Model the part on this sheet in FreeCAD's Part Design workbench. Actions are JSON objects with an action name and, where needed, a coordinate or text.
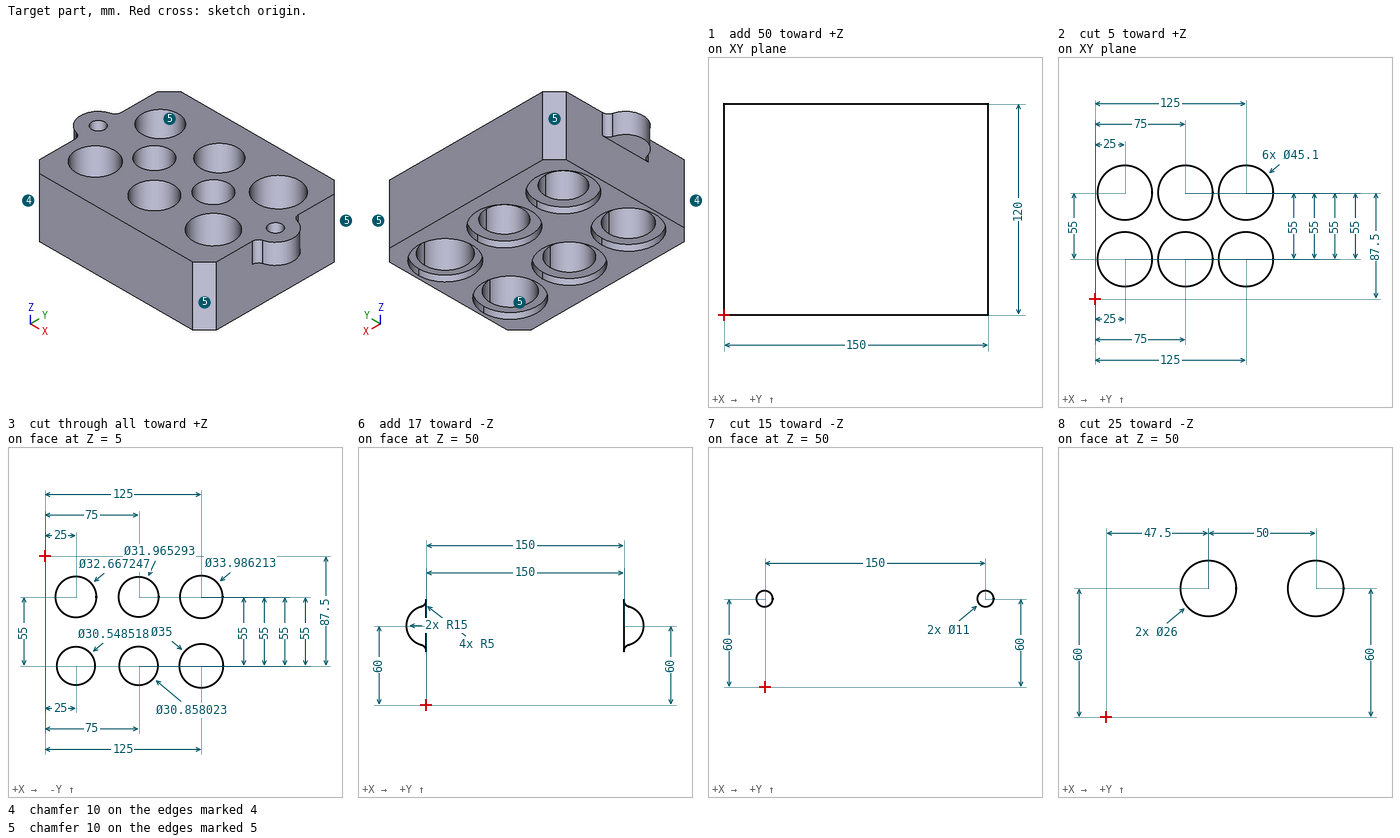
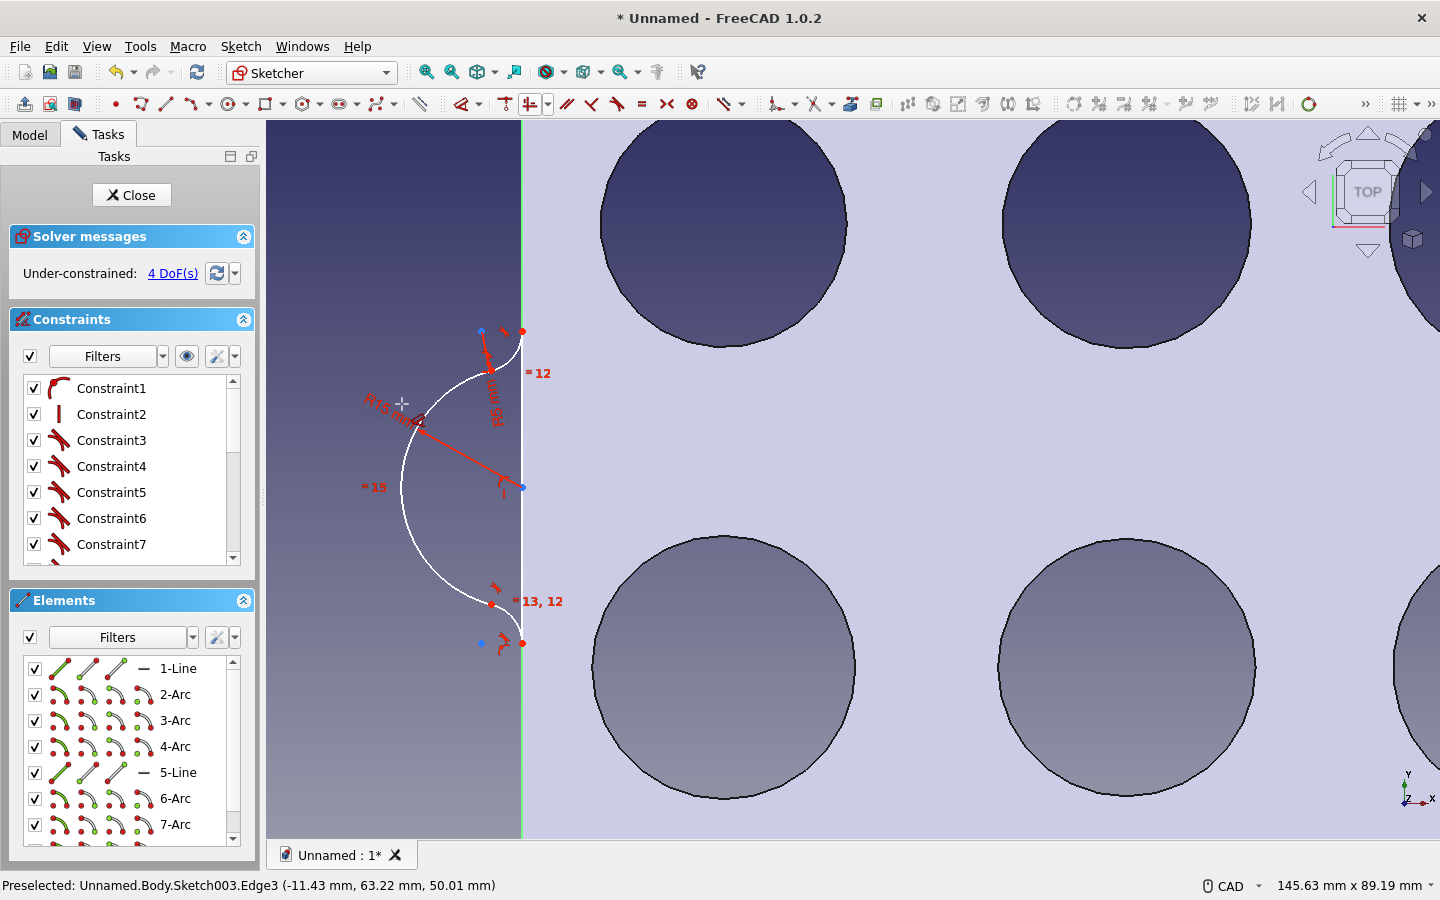
{"action": "left_click", "coordinate": [522, 488]}
{"action": "left_click", "coordinate": [488, 649]}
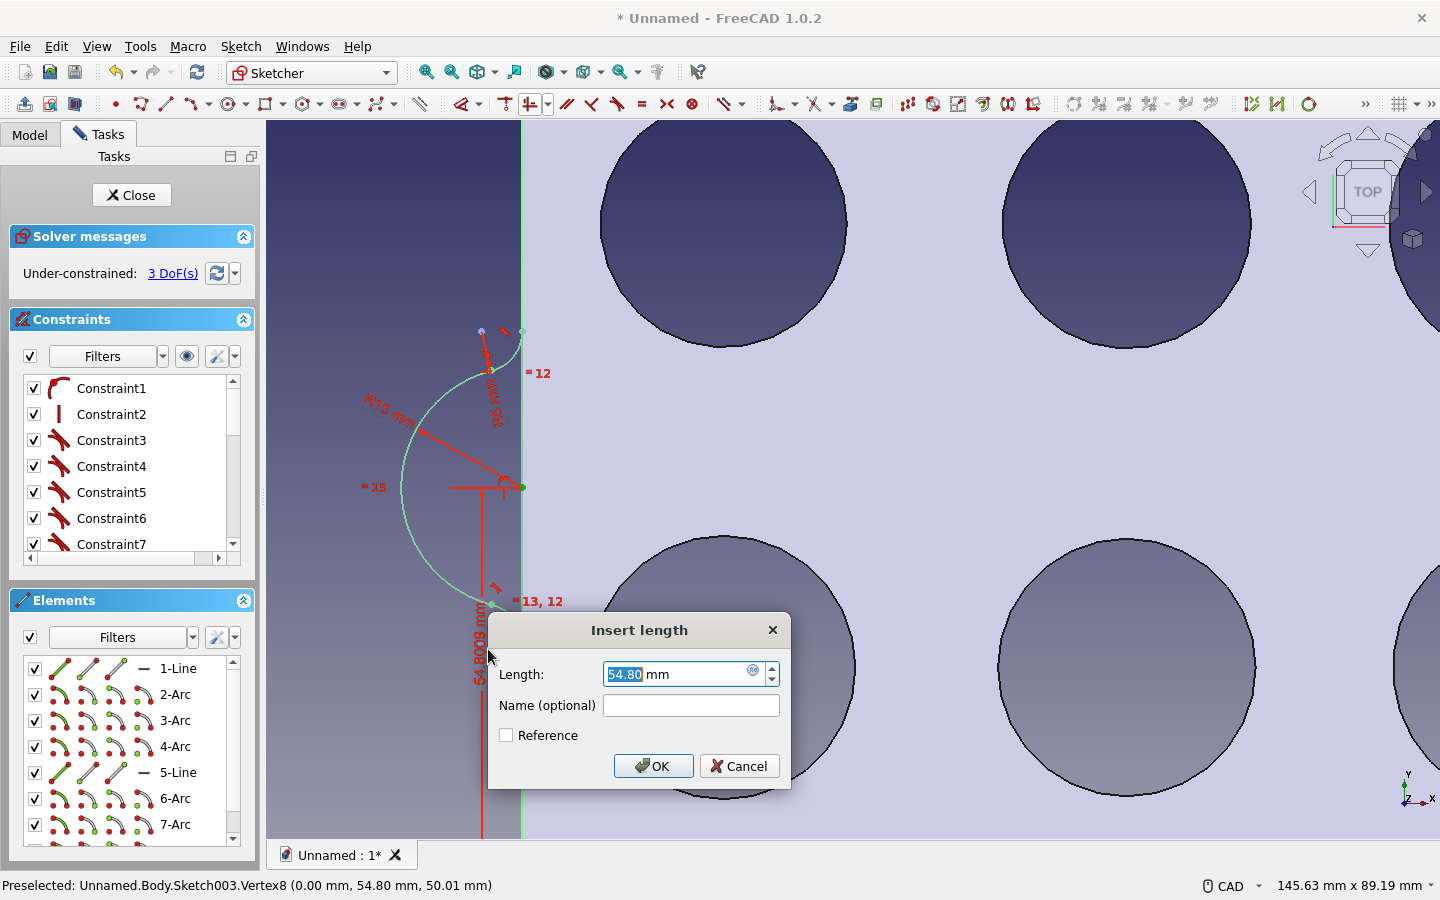
{"action": "type", "text": "60"}
{"action": "key", "text": "Return"}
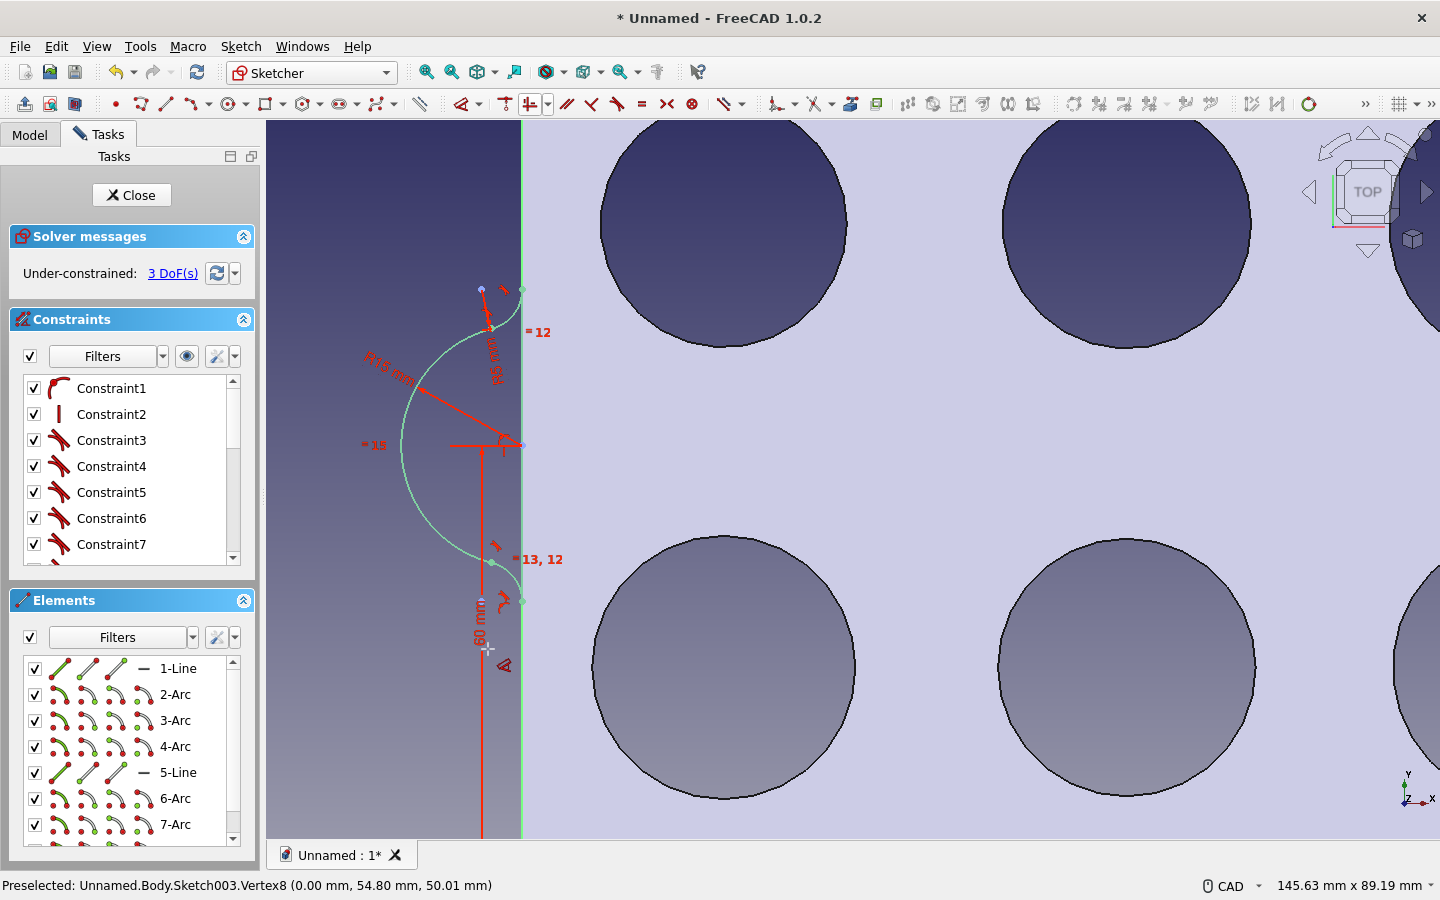
{"action": "scroll", "coordinate": [505, 373], "scroll_direction": "down", "scroll_amount": 4}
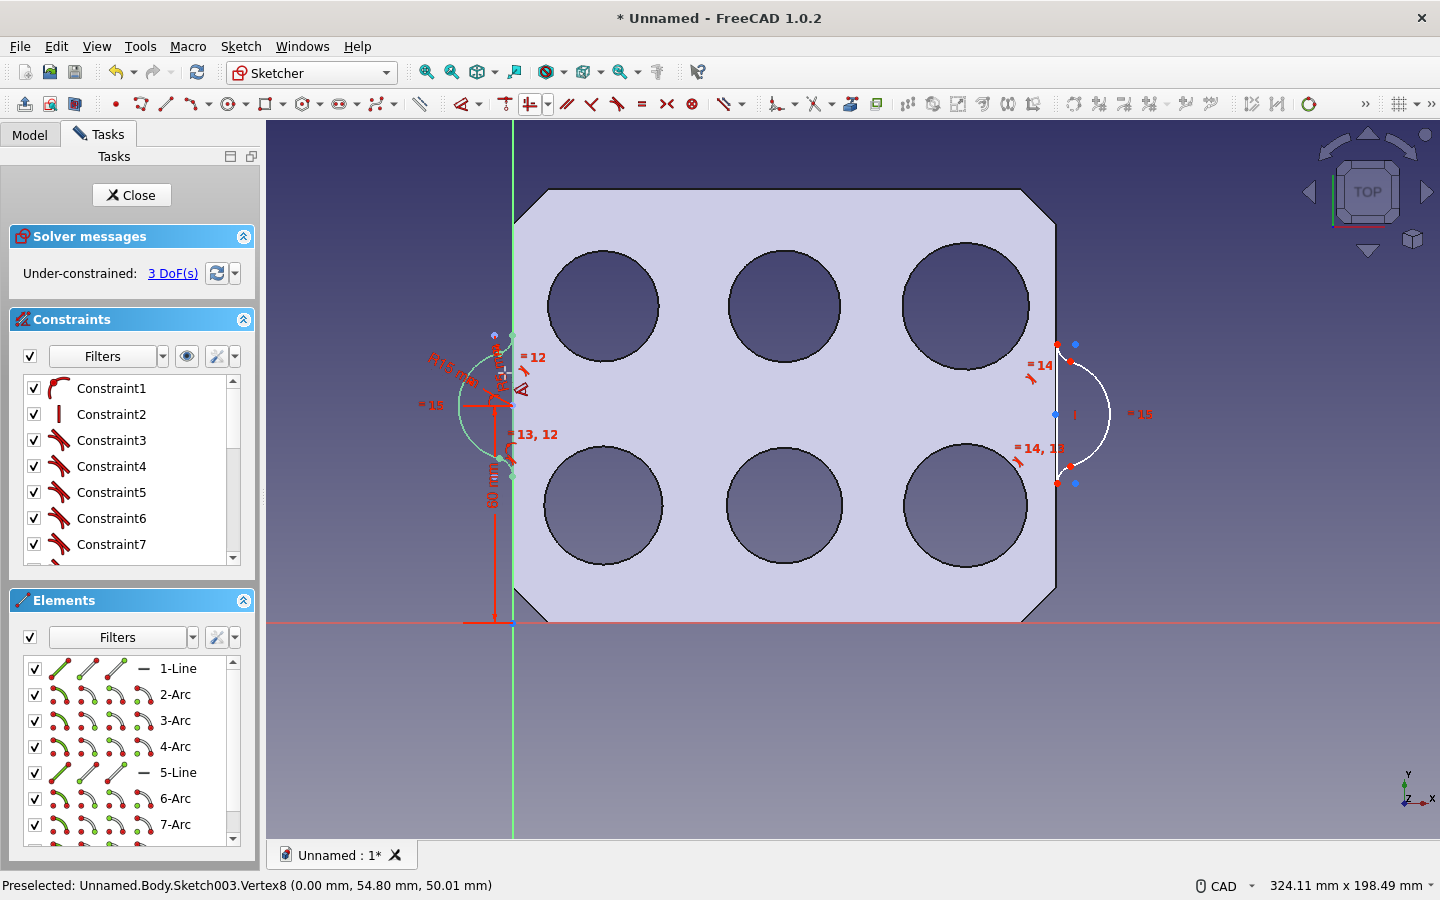
{"action": "left_click", "coordinate": [1055, 414]}
{"action": "left_click", "coordinate": [479, 519]}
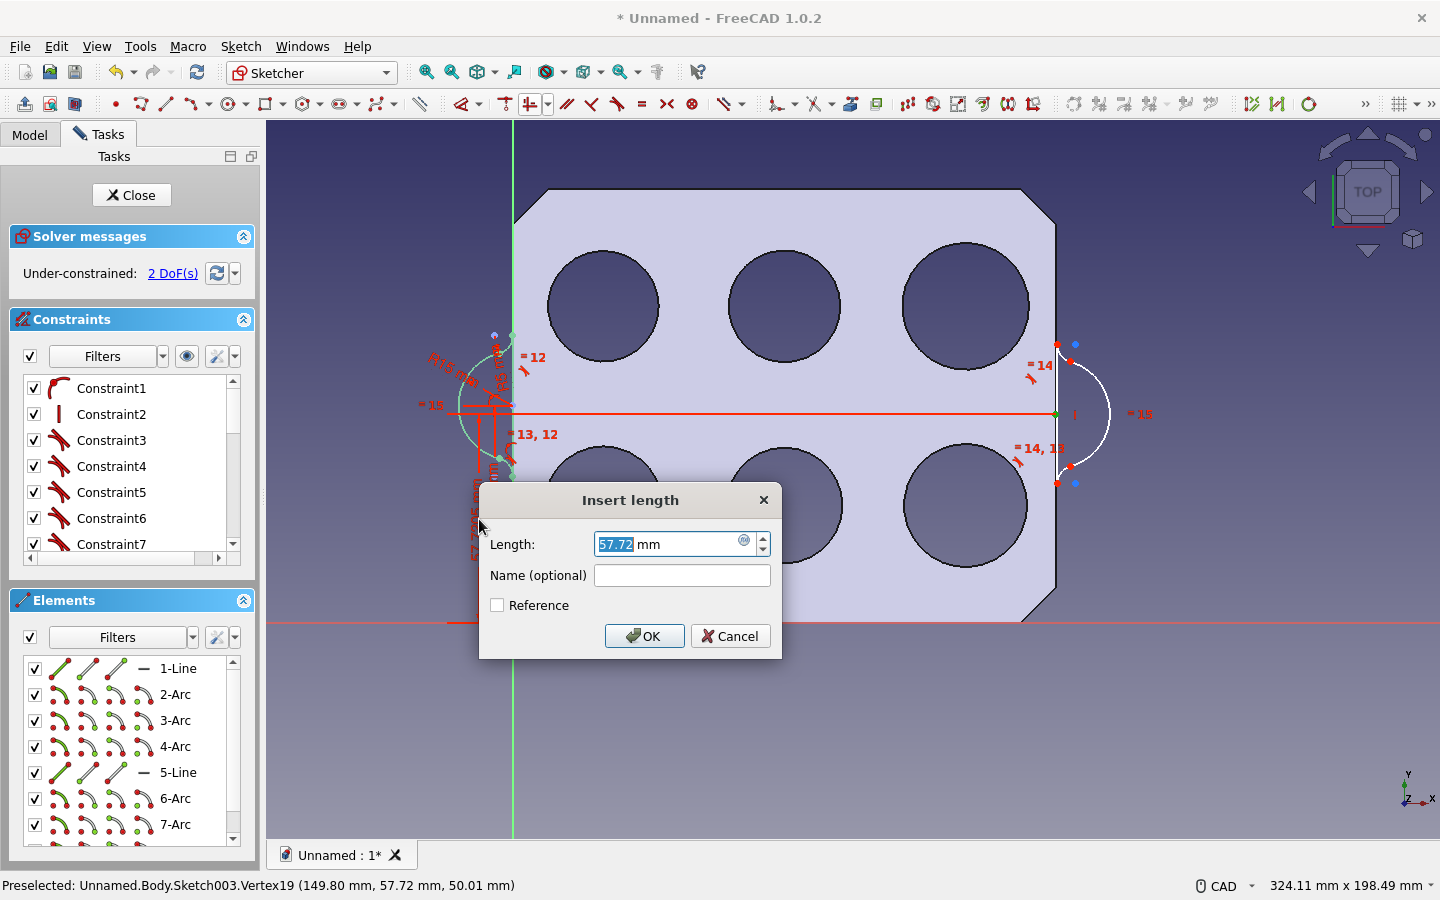
{"action": "type", "text": "60"}
{"action": "key", "text": "Return"}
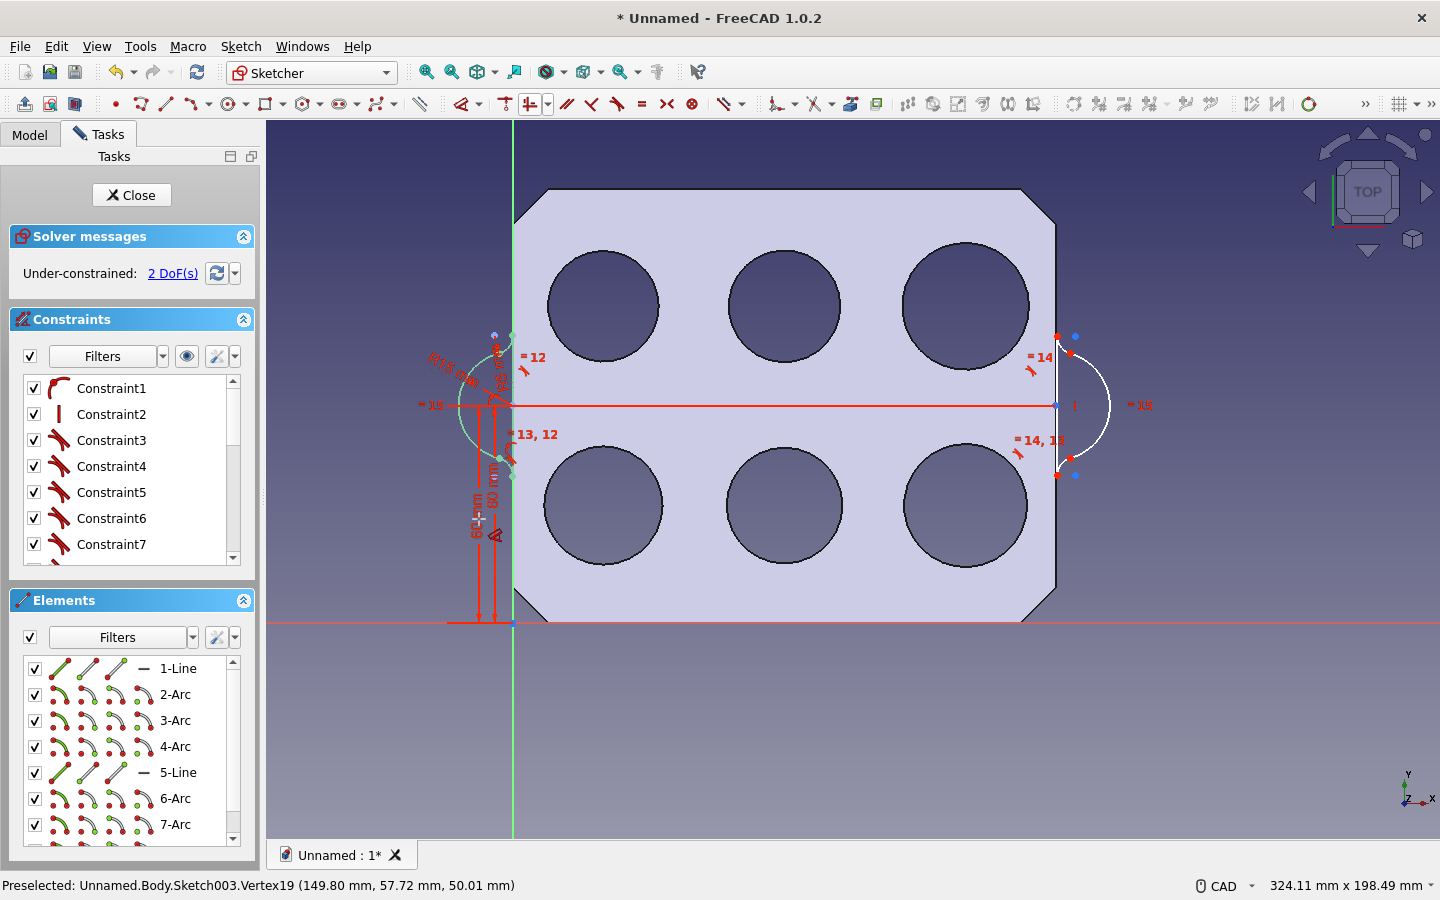
{"action": "left_click", "coordinate": [1057, 336]}
{"action": "left_click", "coordinate": [785, 657]}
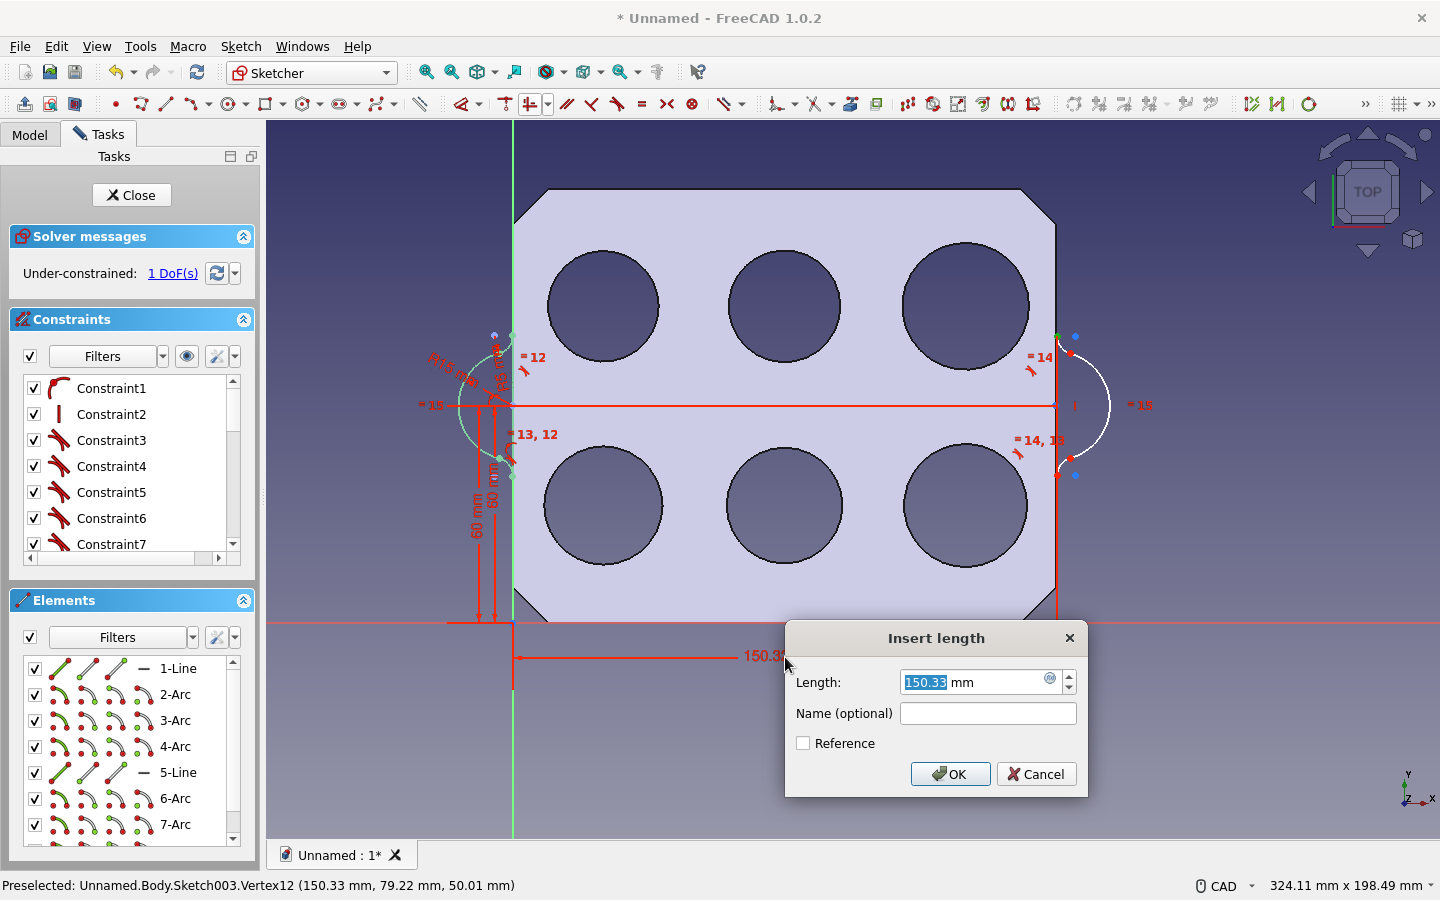
{"action": "type", "text": "150"}
{"action": "key", "text": "Return"}